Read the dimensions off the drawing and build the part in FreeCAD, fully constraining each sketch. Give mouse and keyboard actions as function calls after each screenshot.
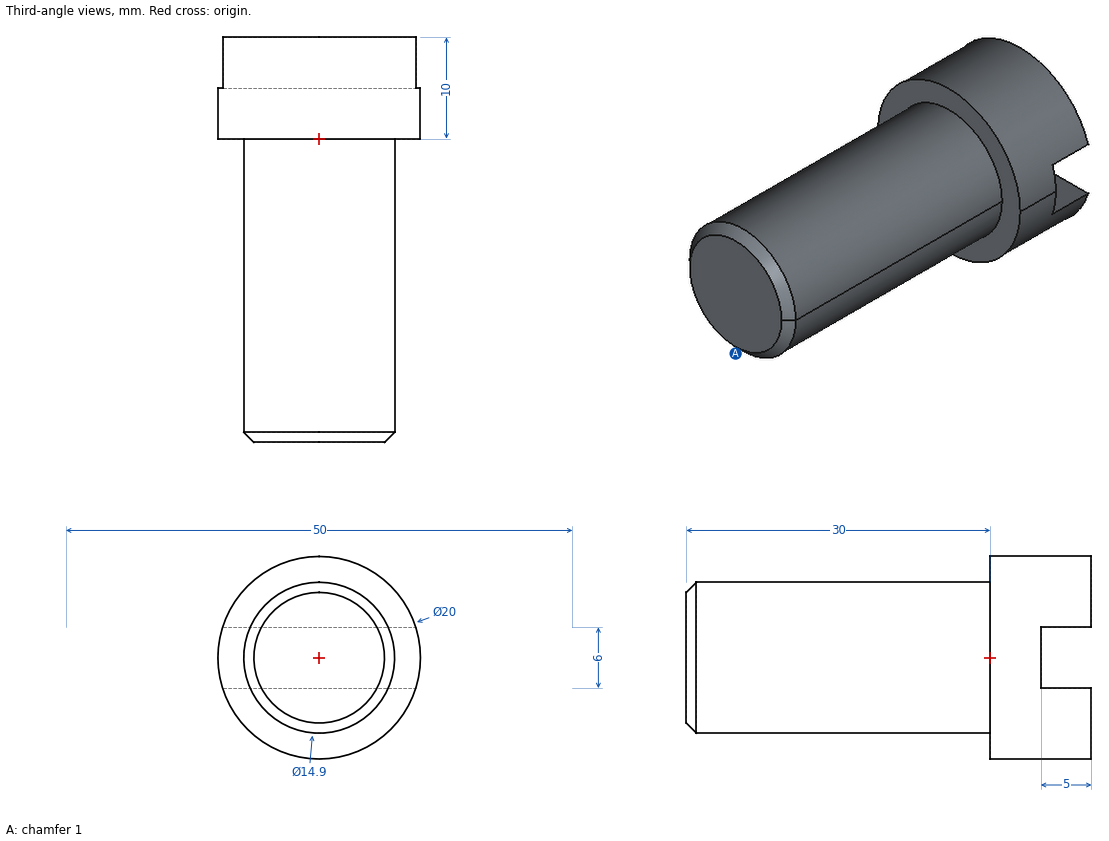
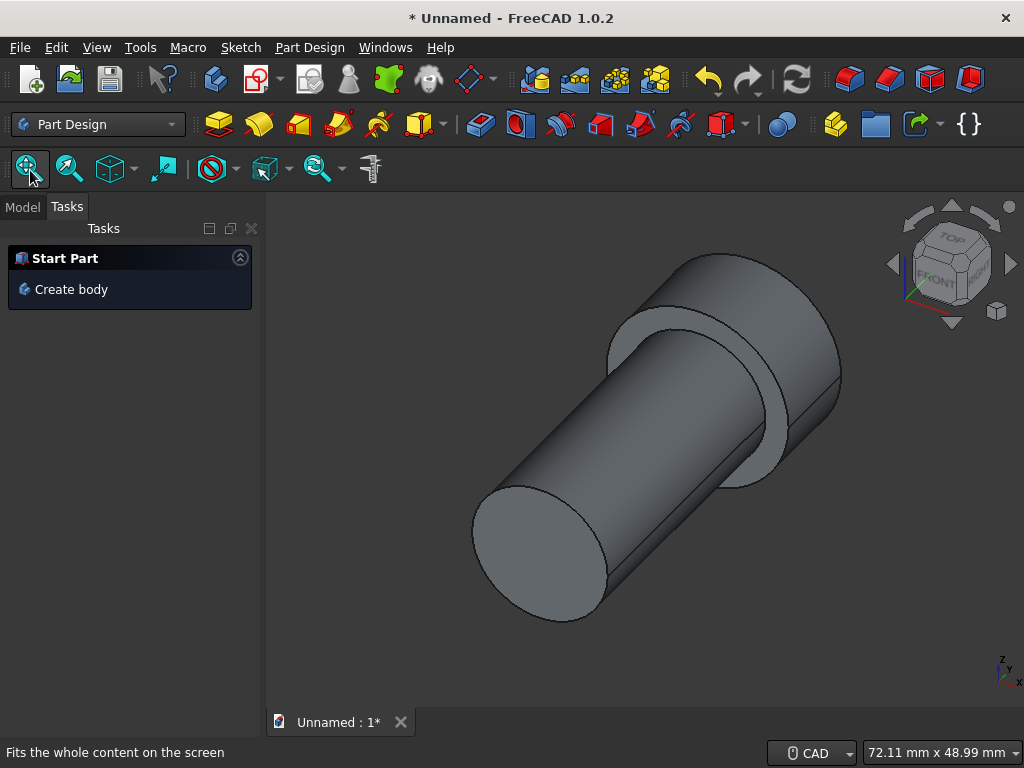
key(4)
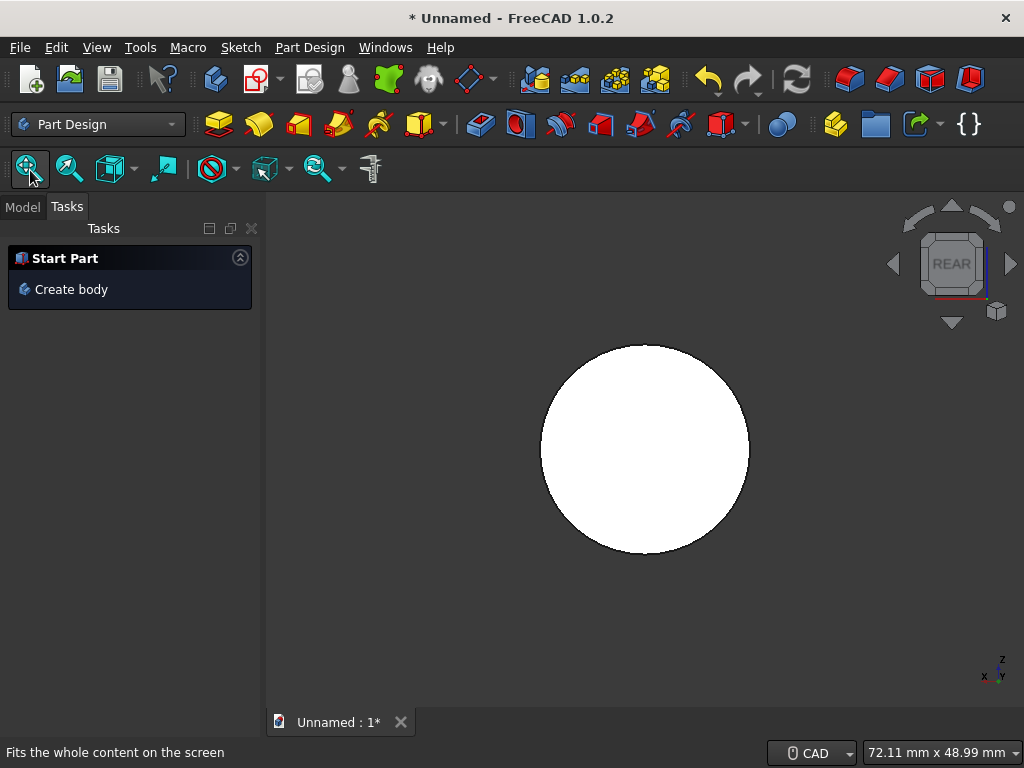
click(30, 170)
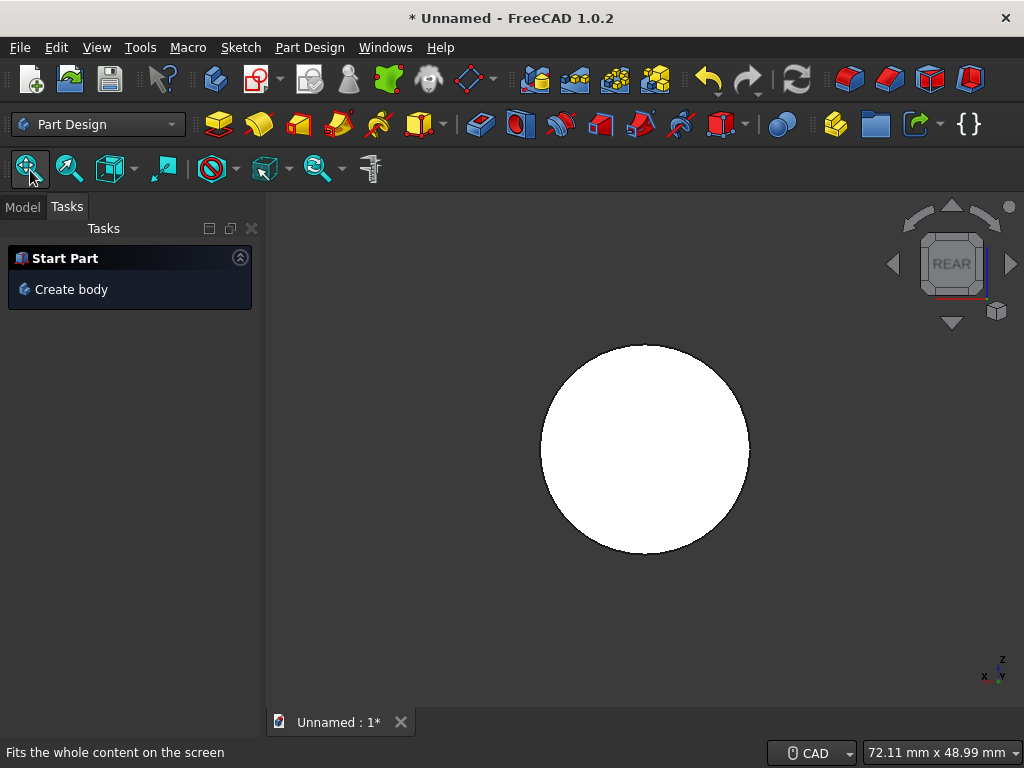
click(645, 448)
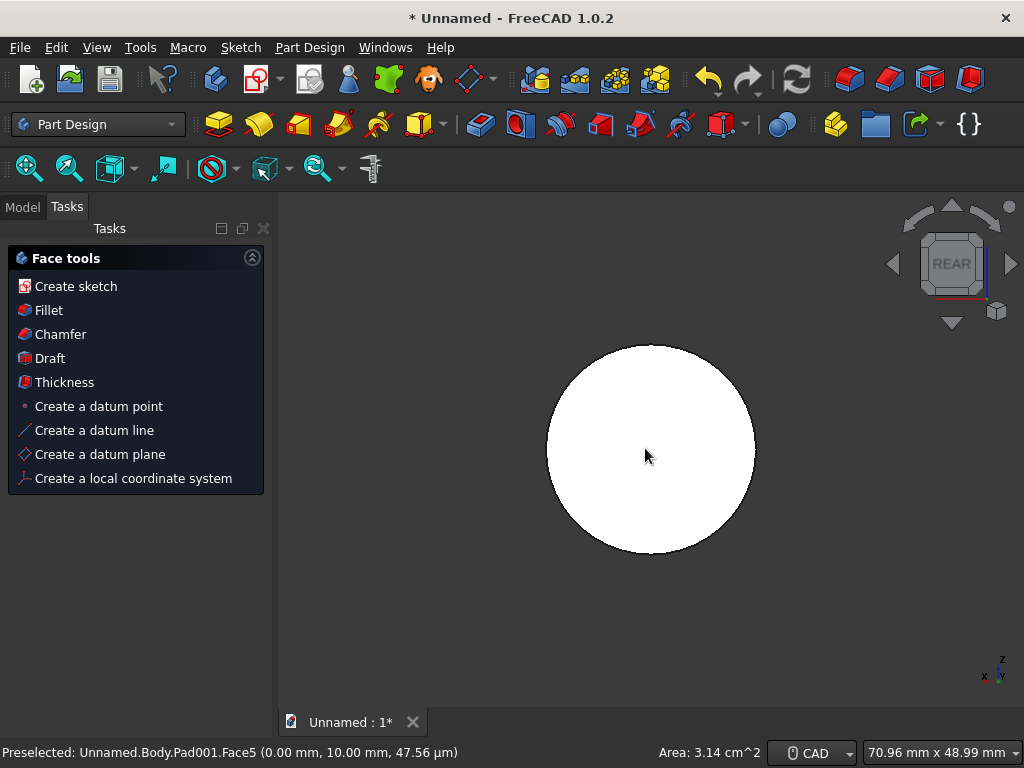
click(256, 80)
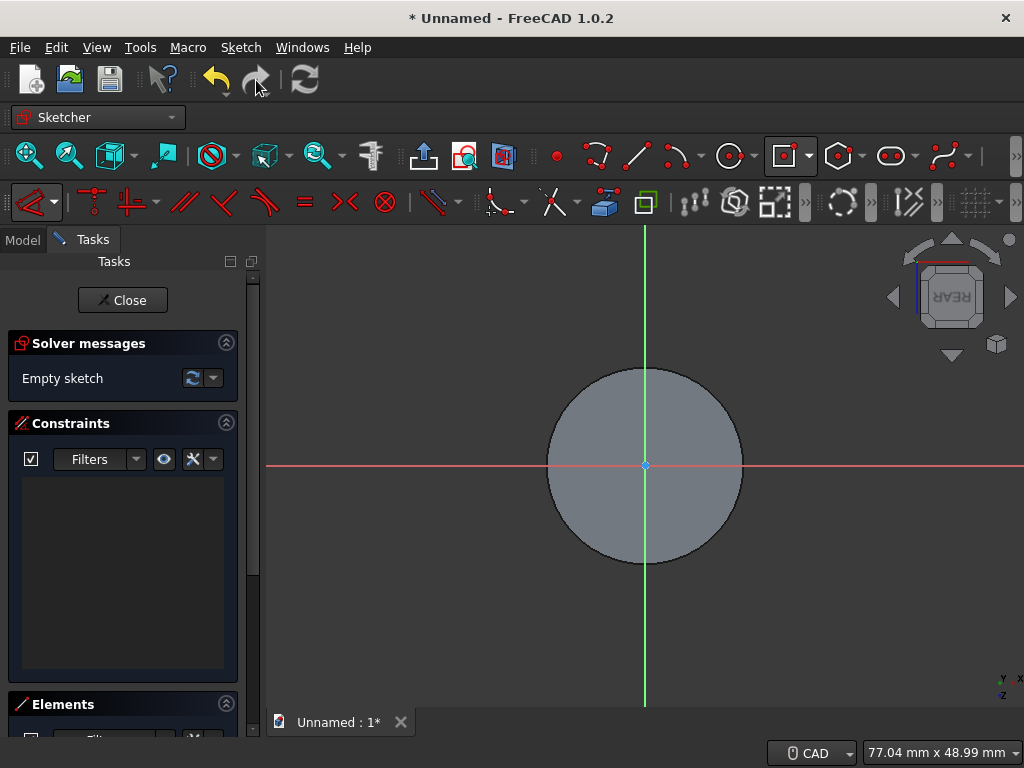
scroll(294, 466, down, 1)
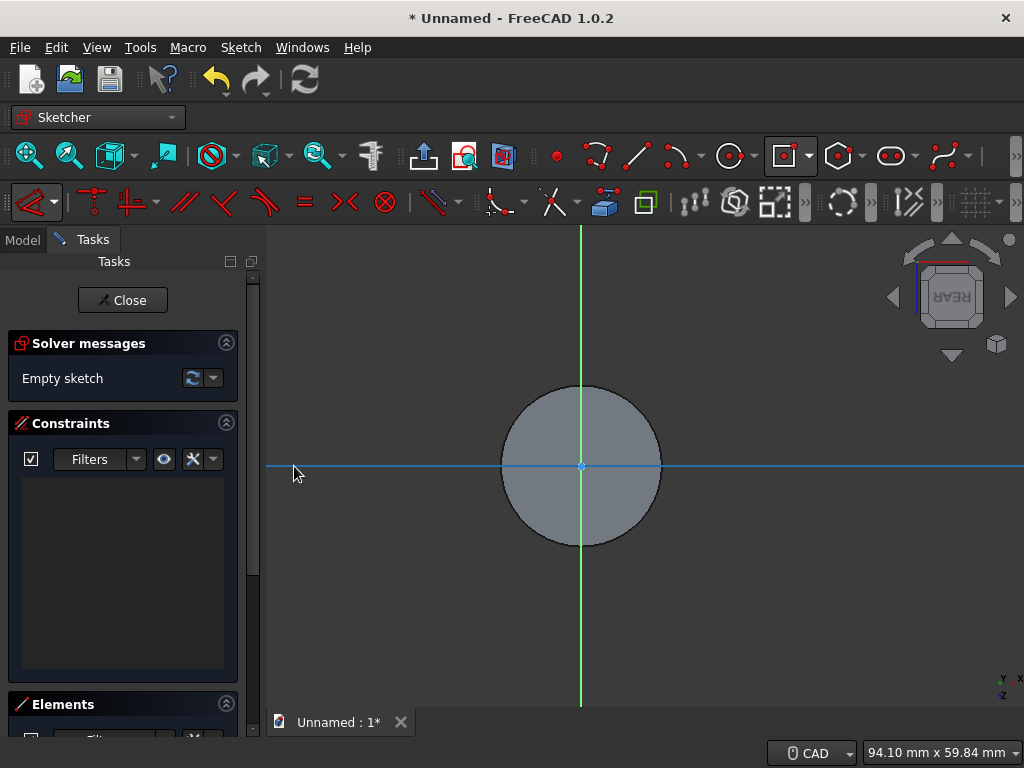
click(784, 156)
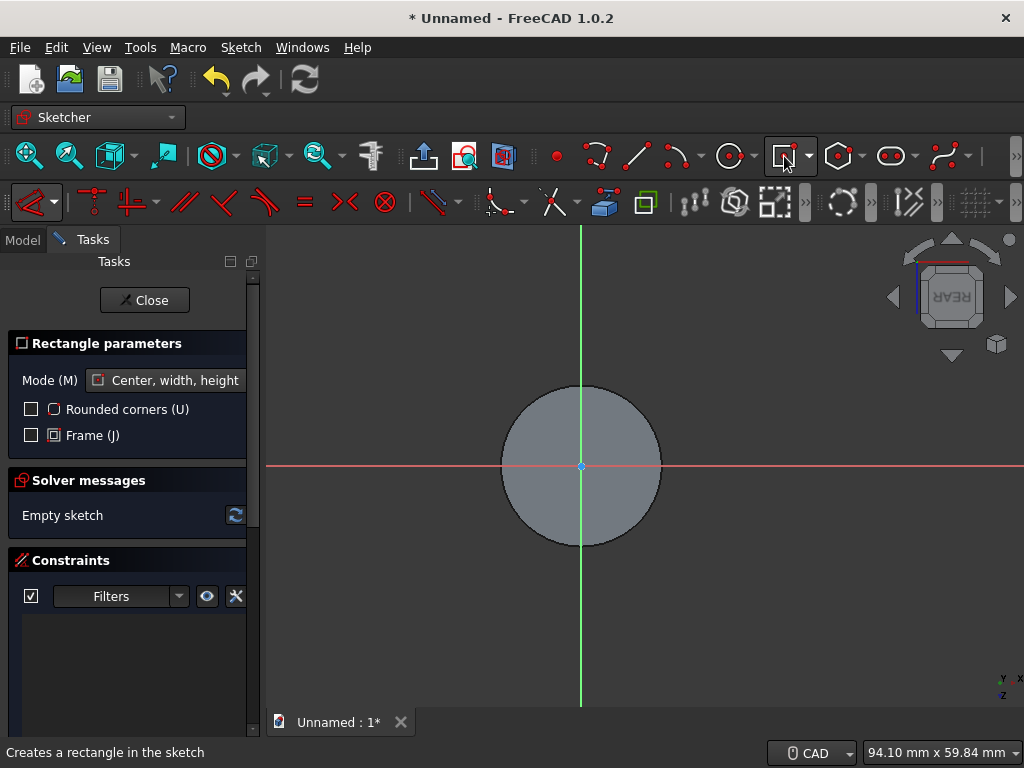
click(581, 466)
move(783, 442)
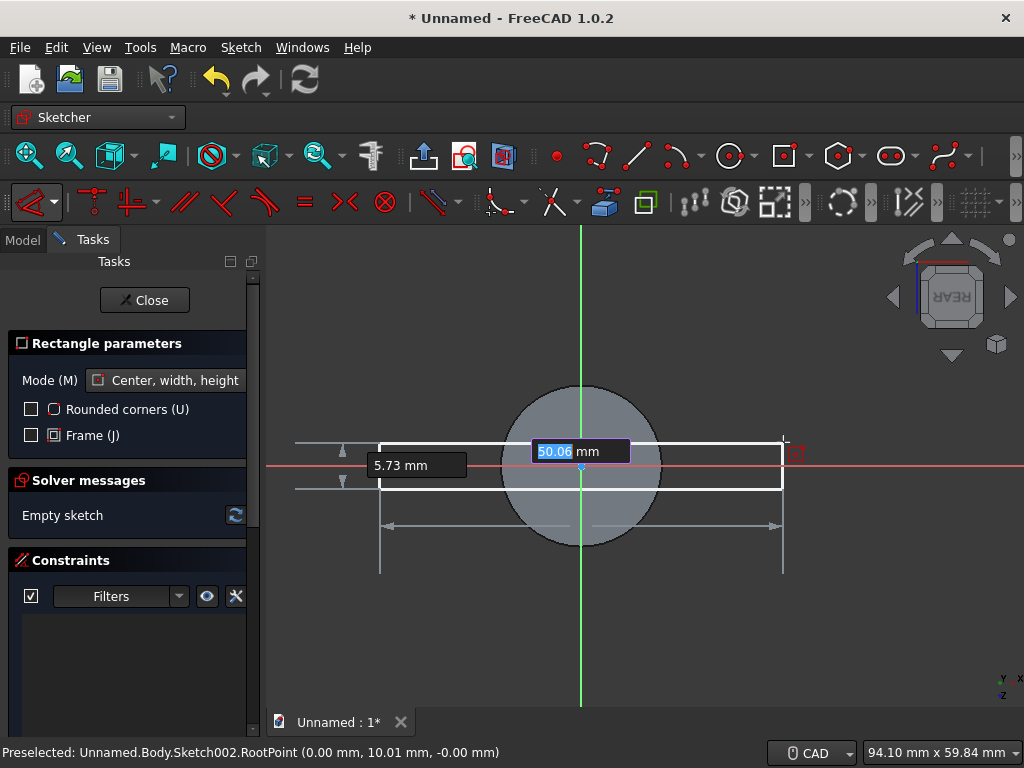
text(50)
key(Tab)
text(6)
key(Return)
key(Escape)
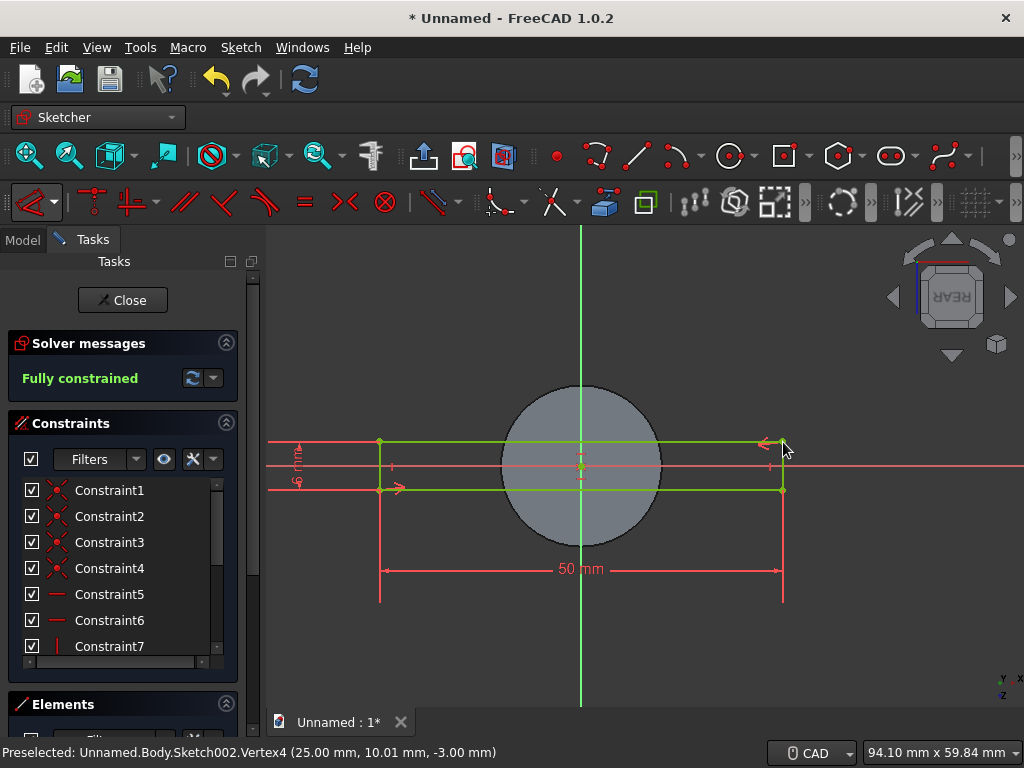
click(123, 300)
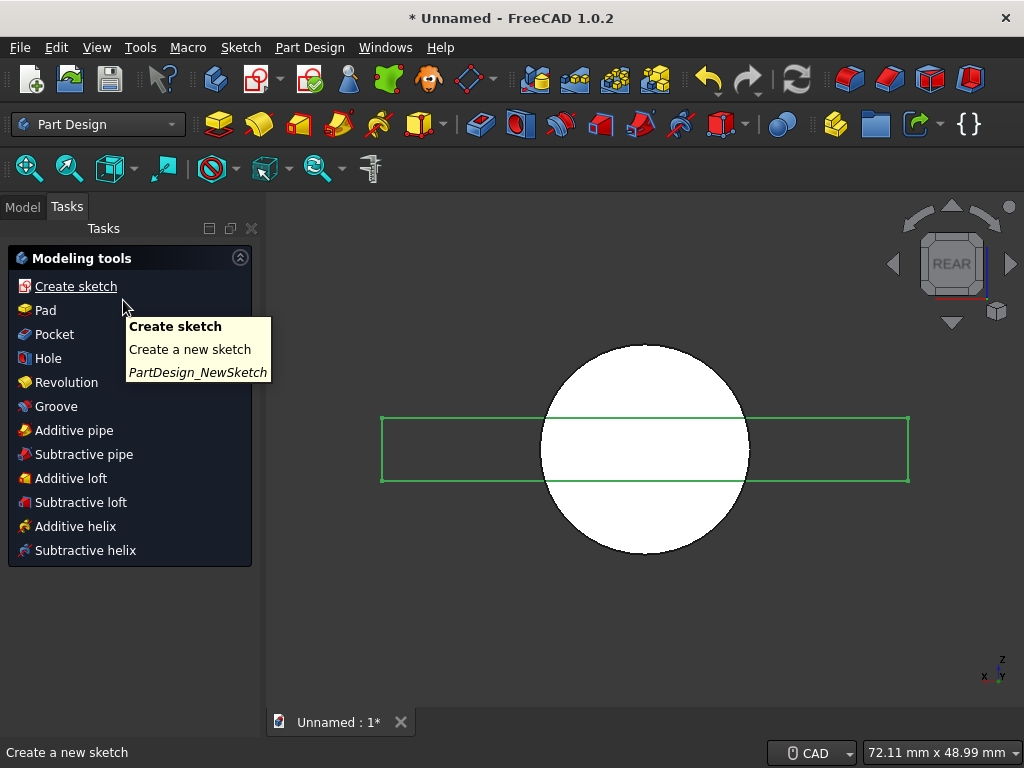
click(482, 124)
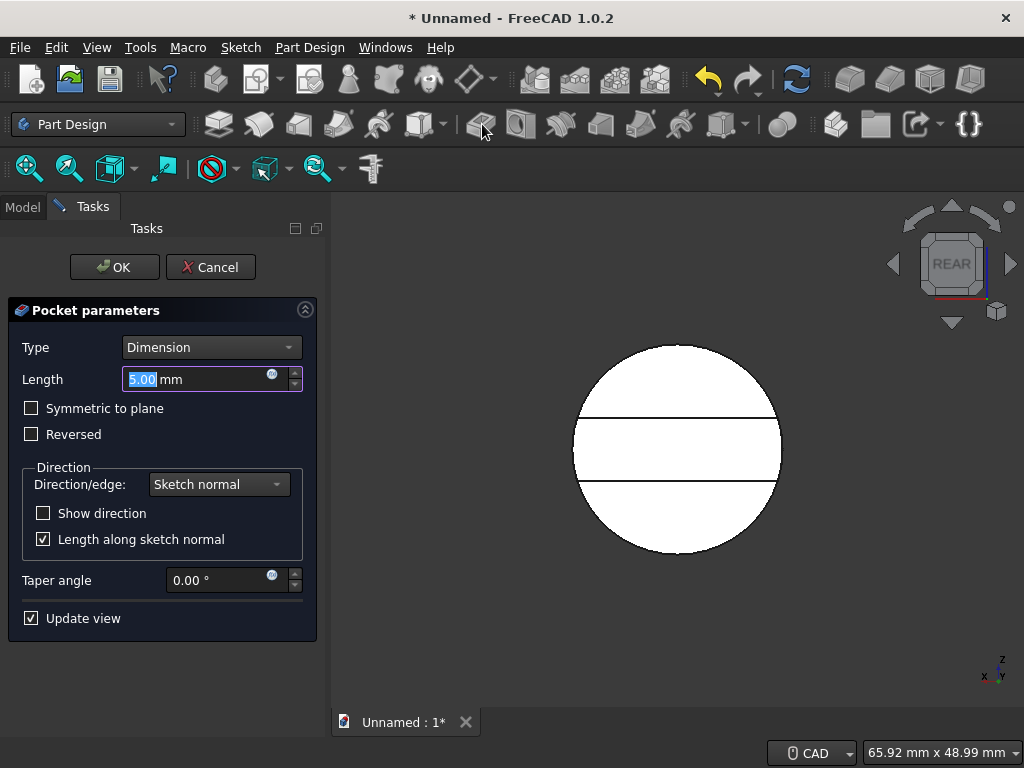
text(5)
key(Tab)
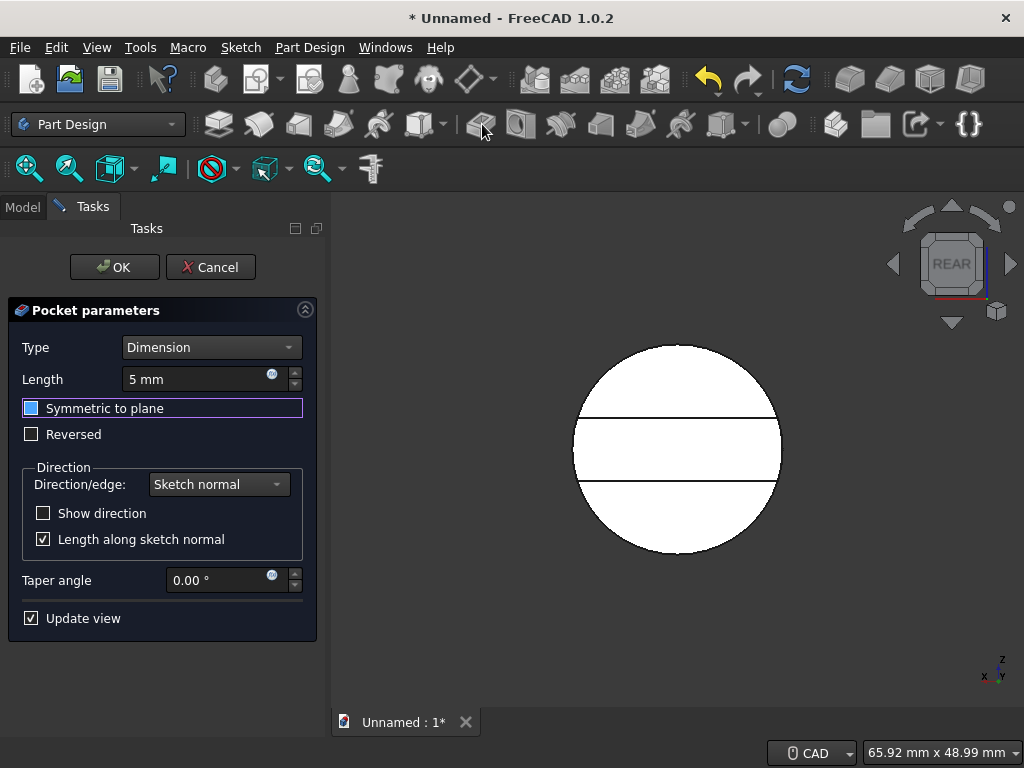
click(115, 267)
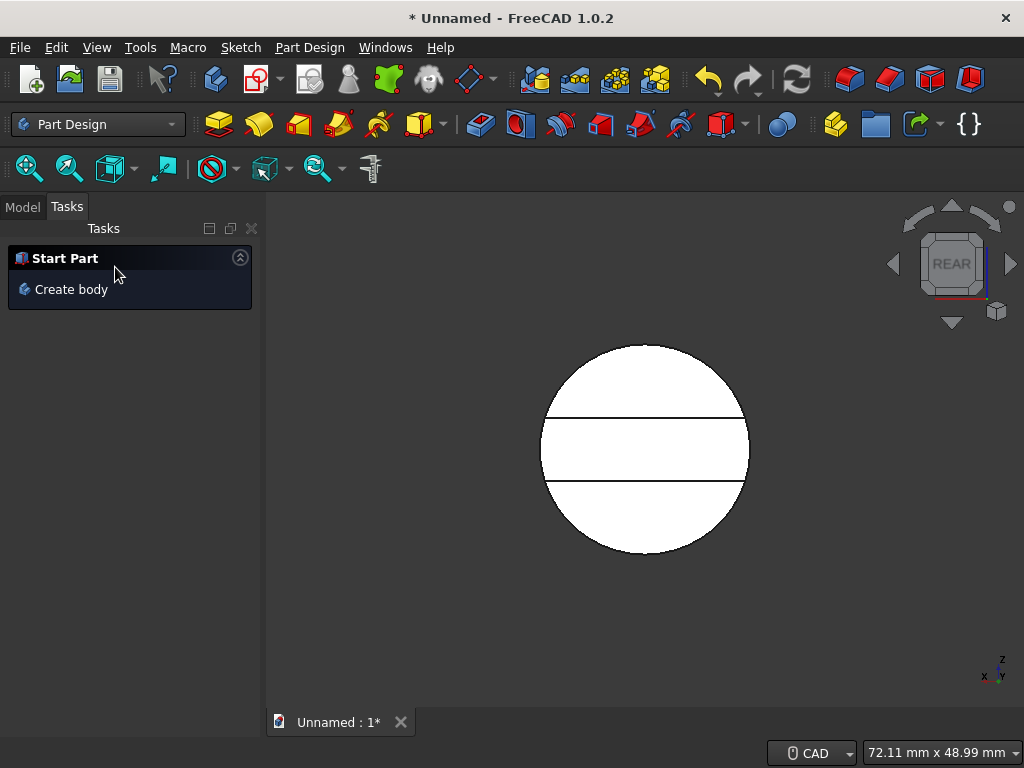
click(30, 170)